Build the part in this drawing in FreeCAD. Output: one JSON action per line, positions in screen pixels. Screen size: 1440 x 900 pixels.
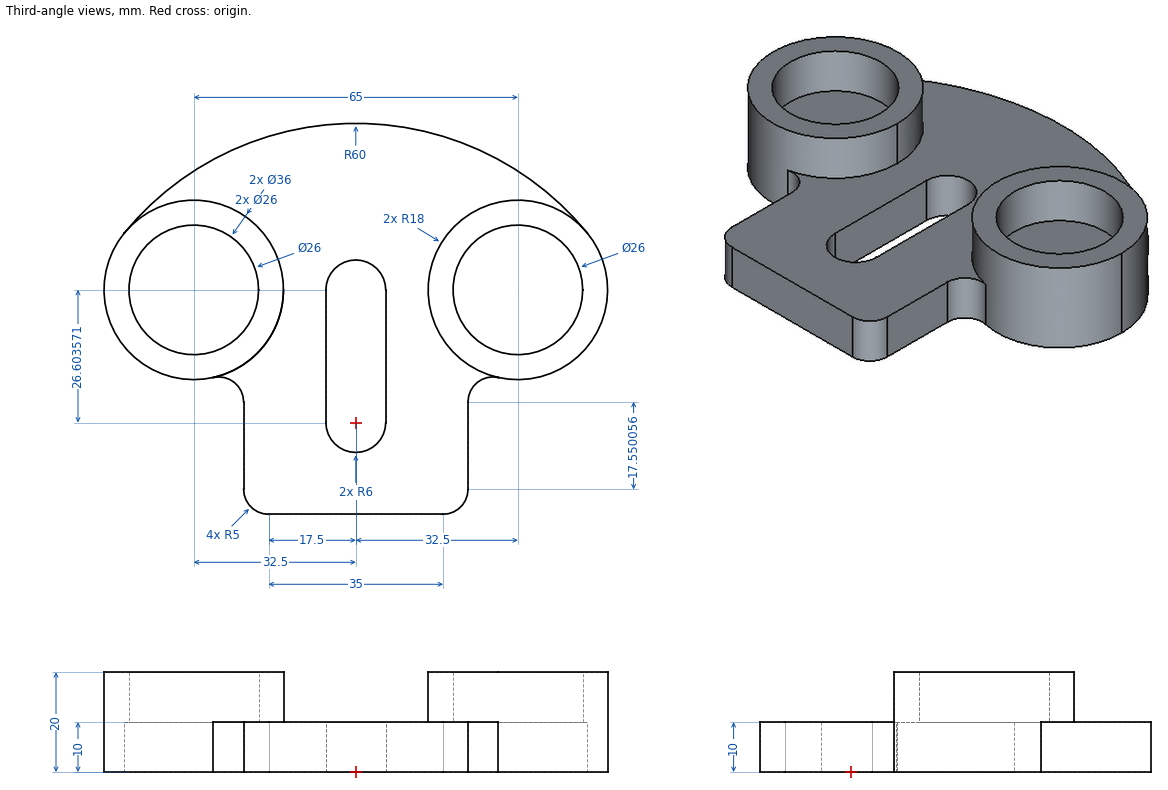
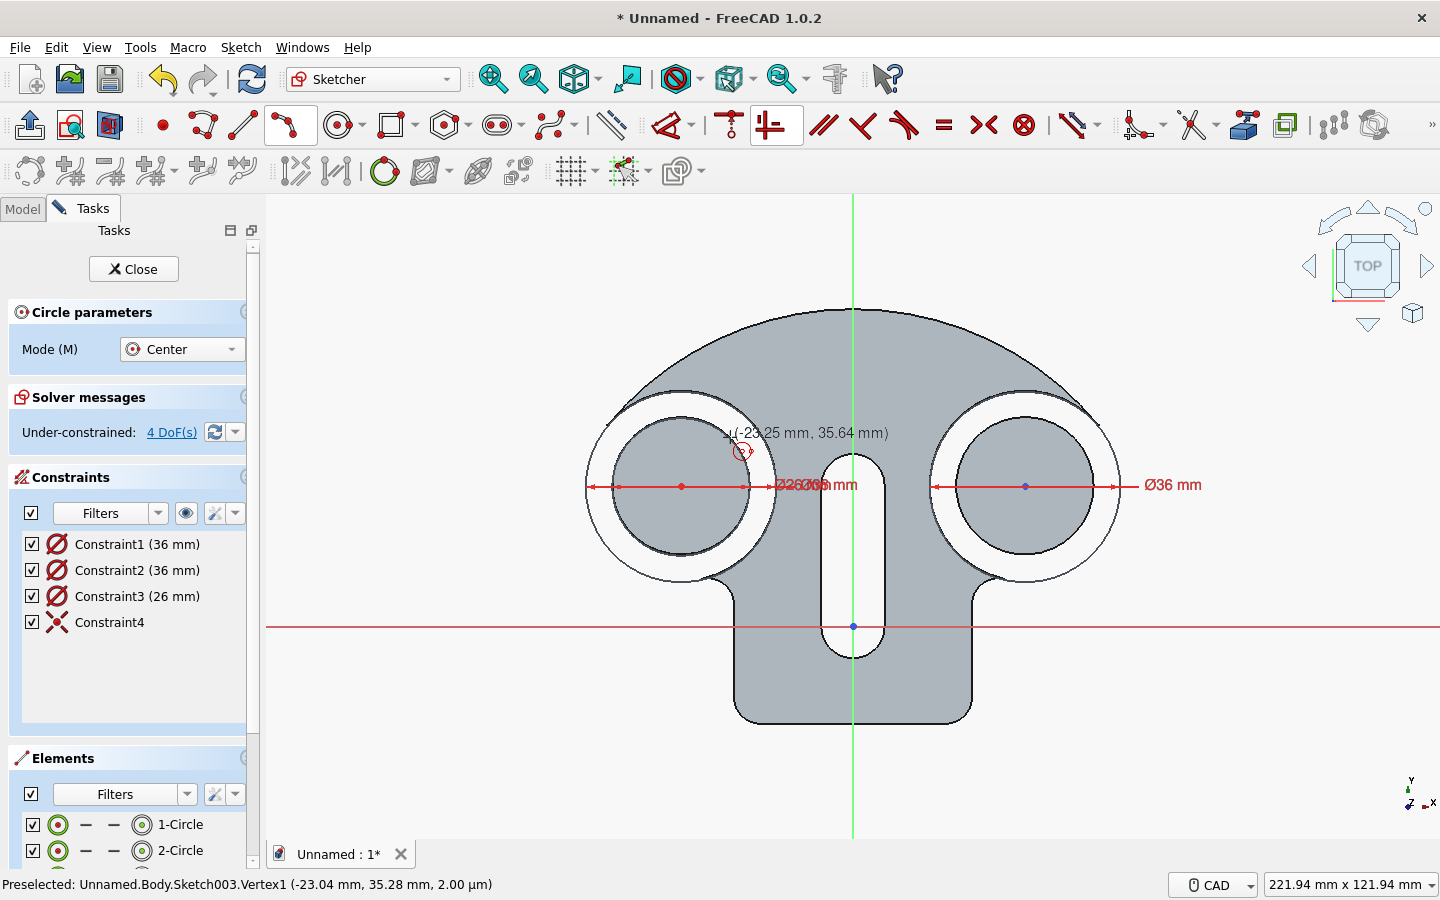
{"action": "left_click", "coordinate": [1025, 487]}
{"action": "mouse_move", "coordinate": [1074, 437]}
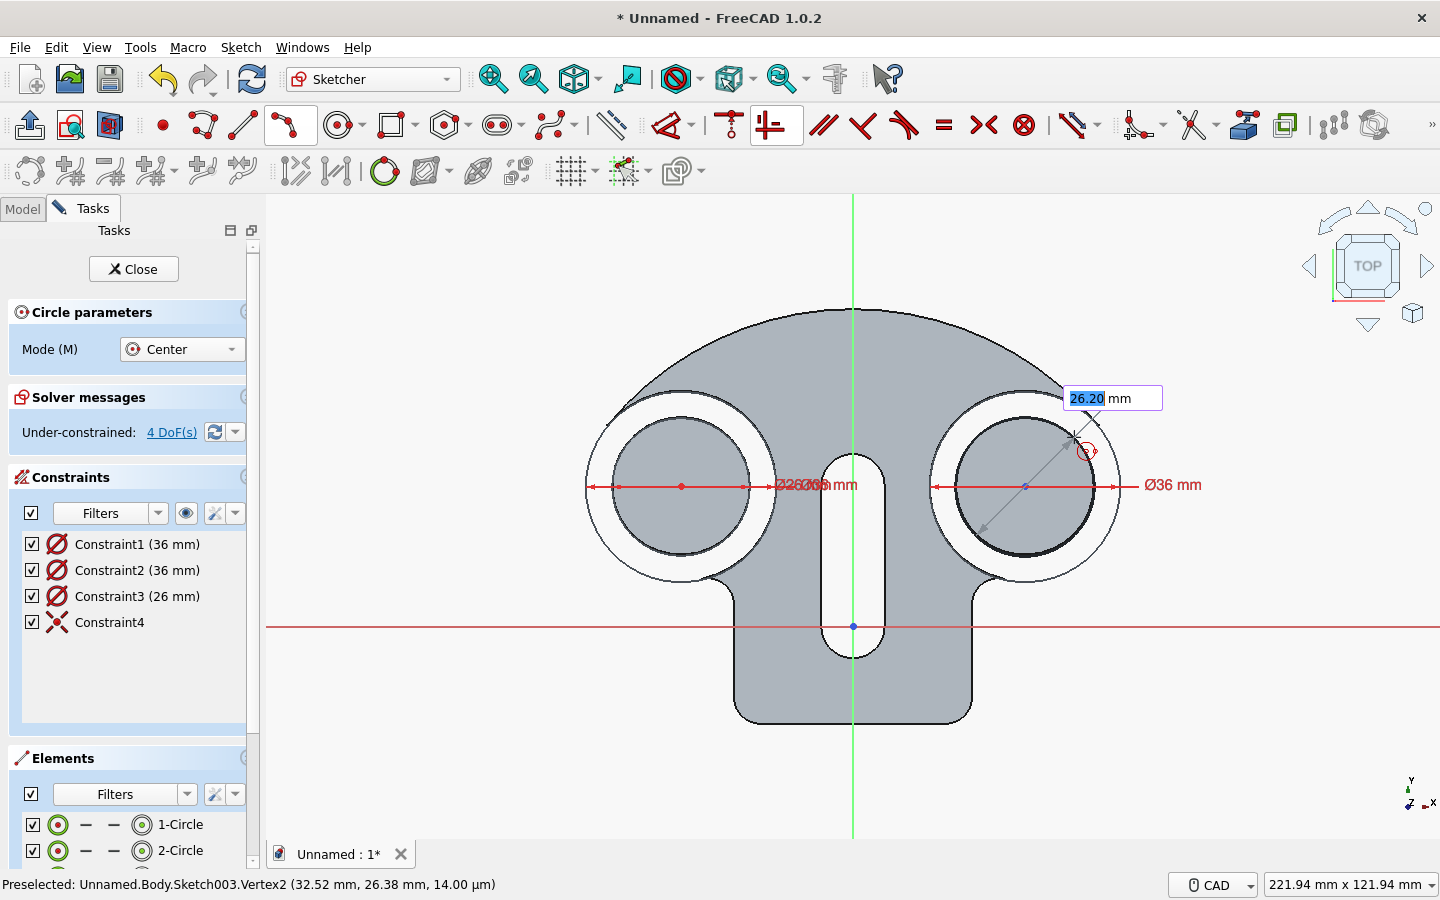
{"action": "type", "text": "26"}
{"action": "key", "text": "Return"}
{"action": "key", "text": "Escape"}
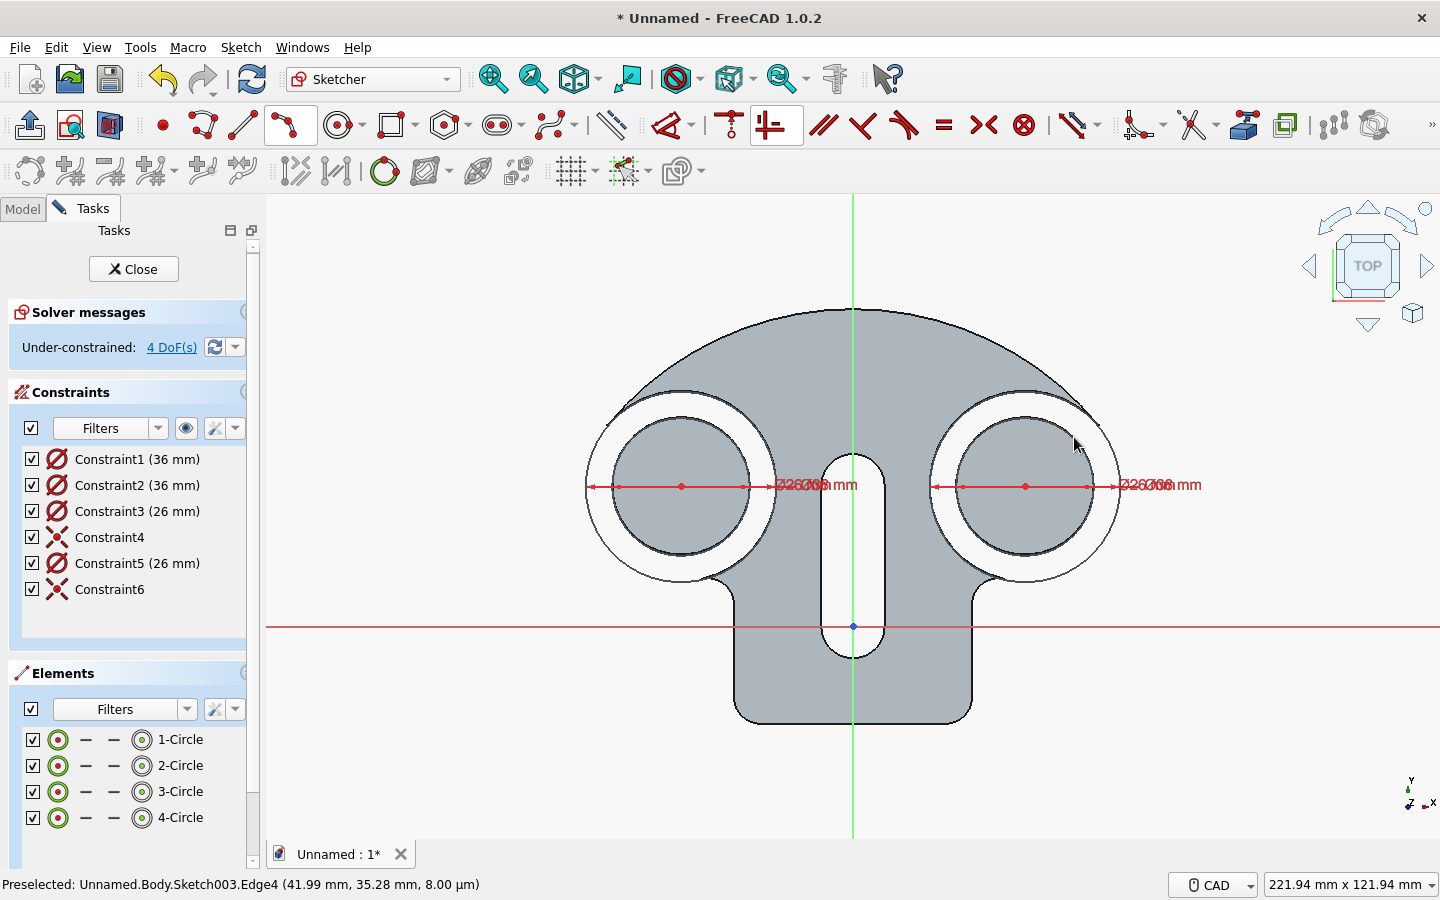
{"action": "left_click", "coordinate": [681, 487]}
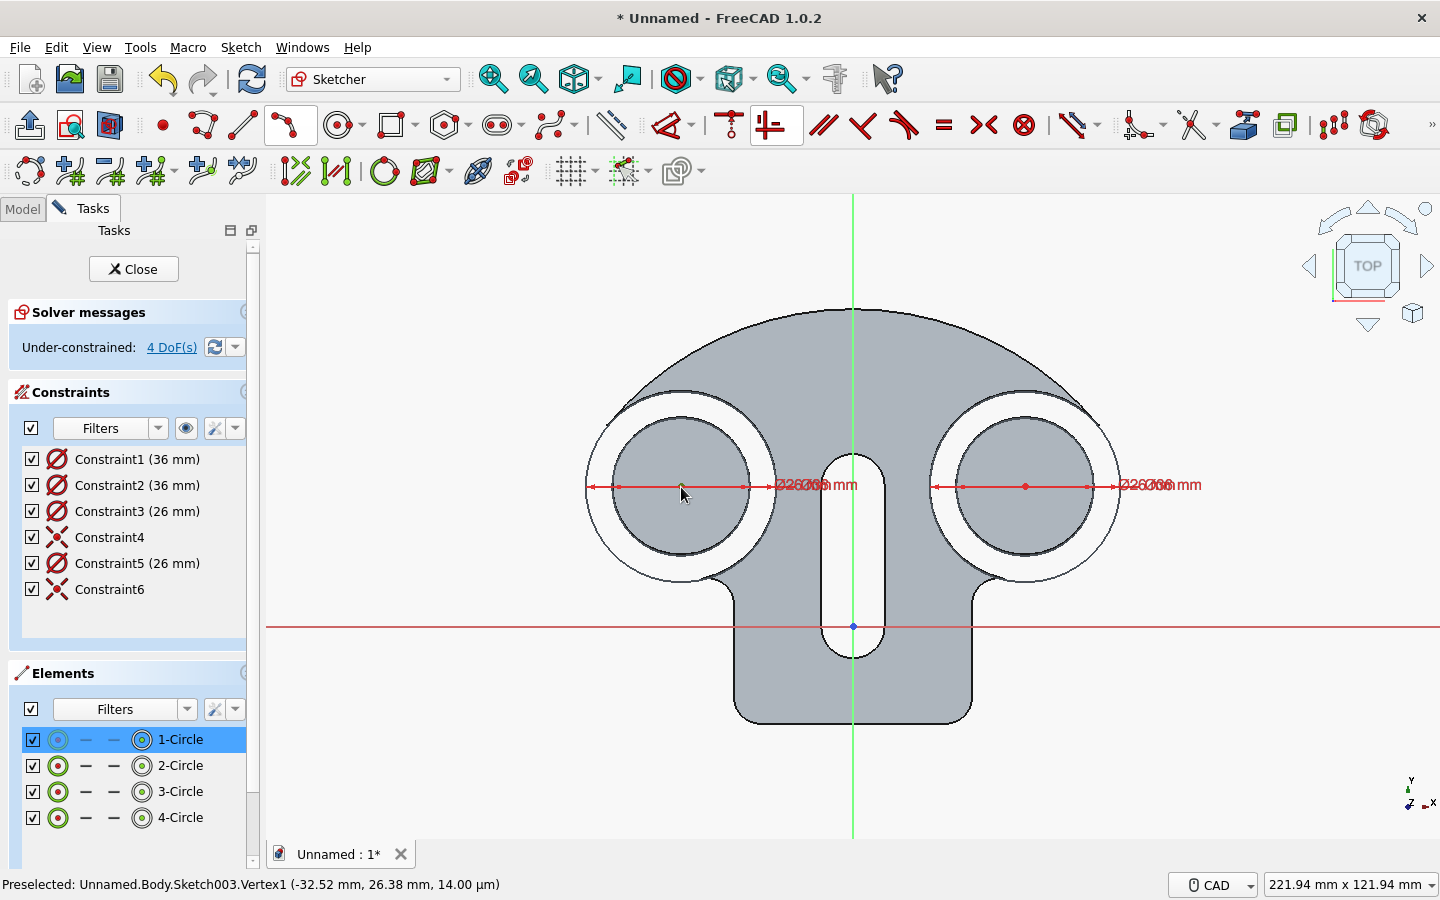
{"action": "left_click", "coordinate": [1025, 487]}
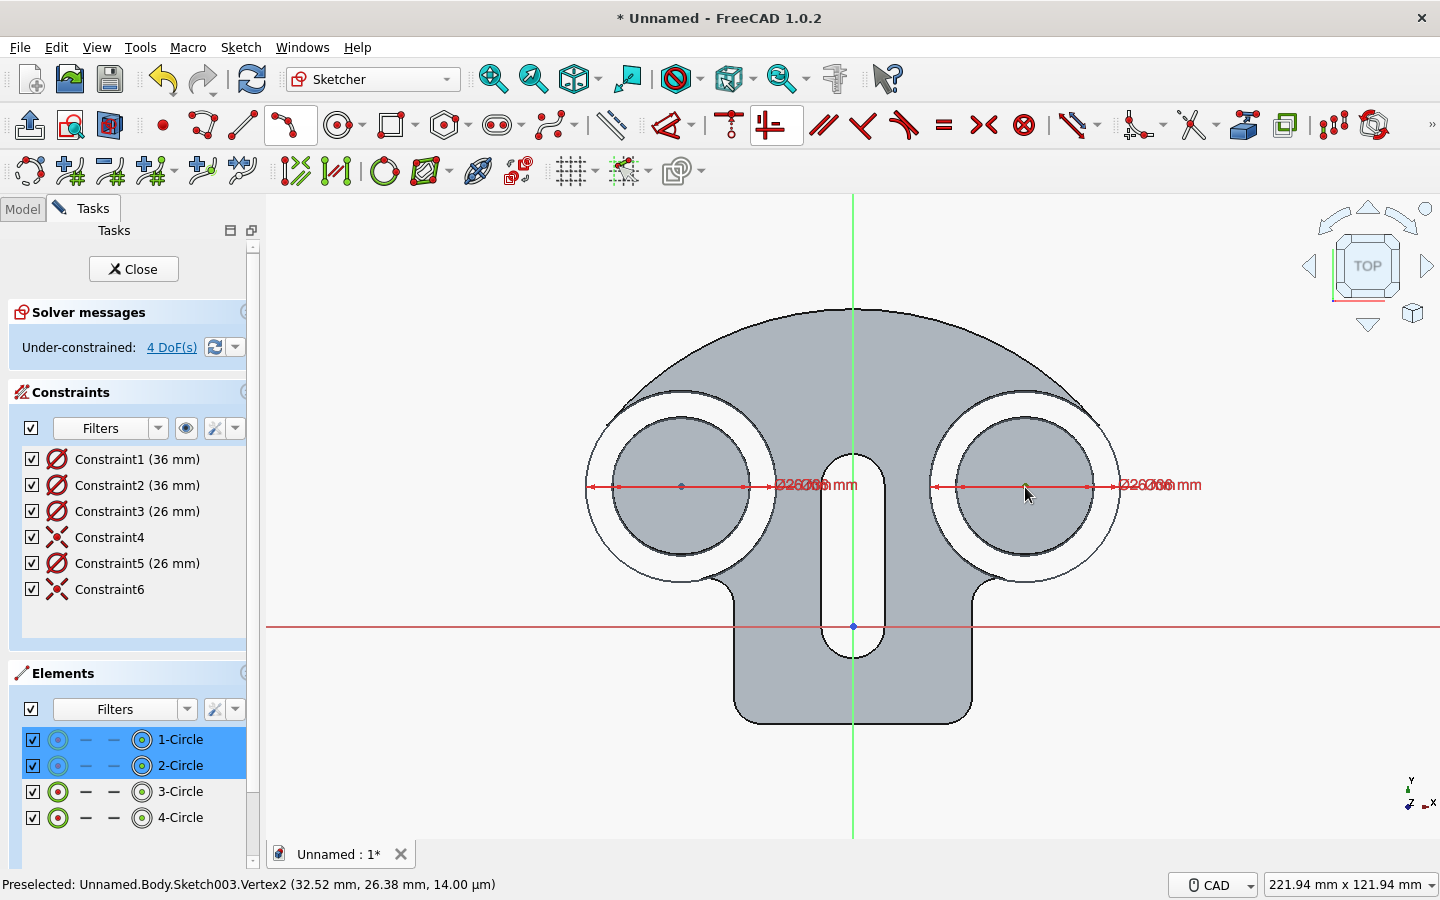
{"action": "key", "text": "h"}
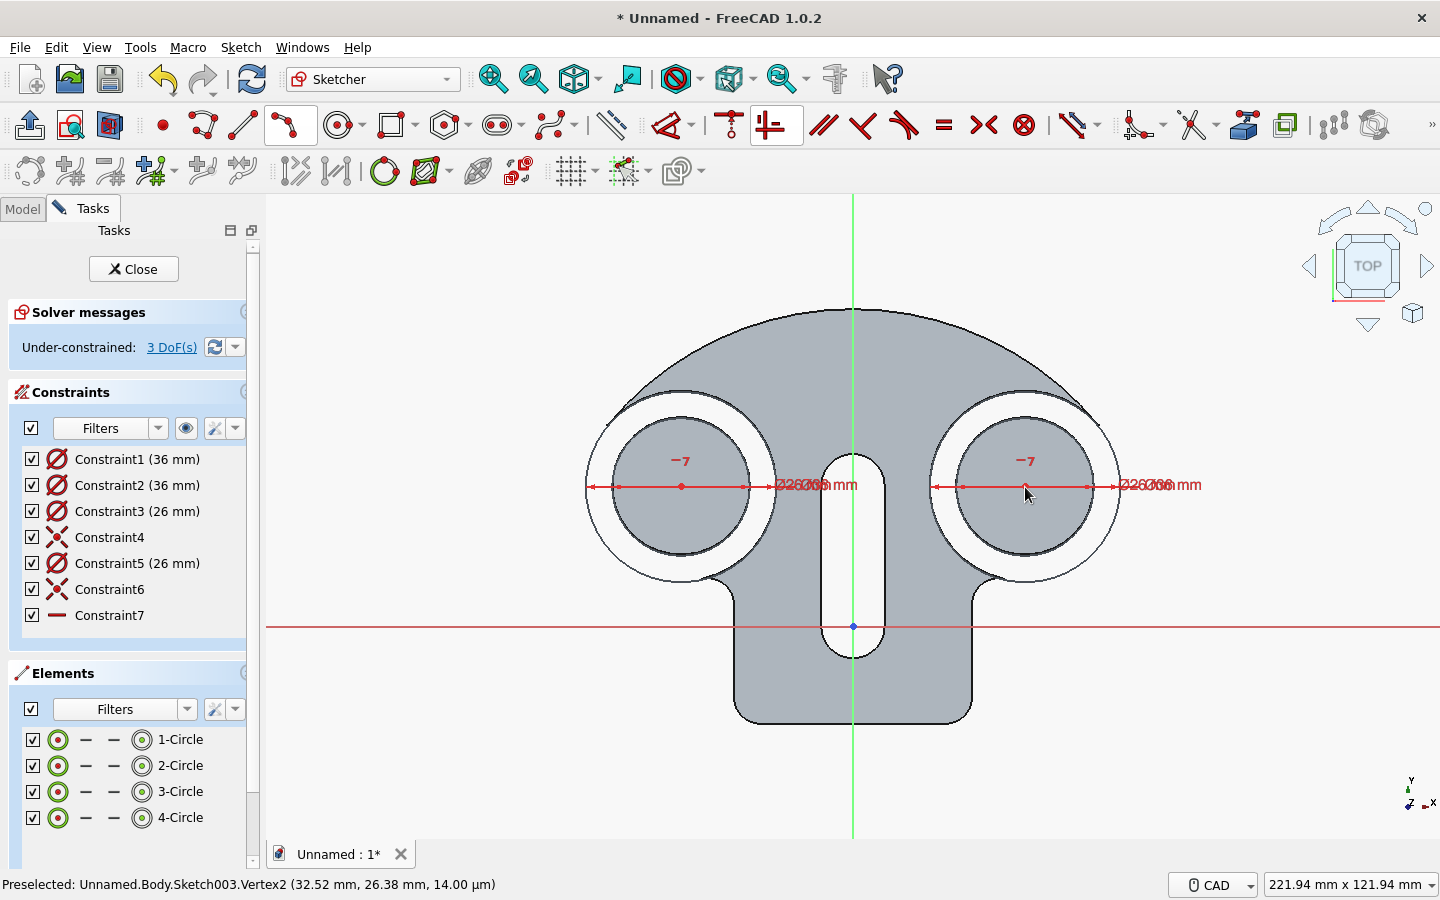
{"action": "left_click", "coordinate": [666, 126]}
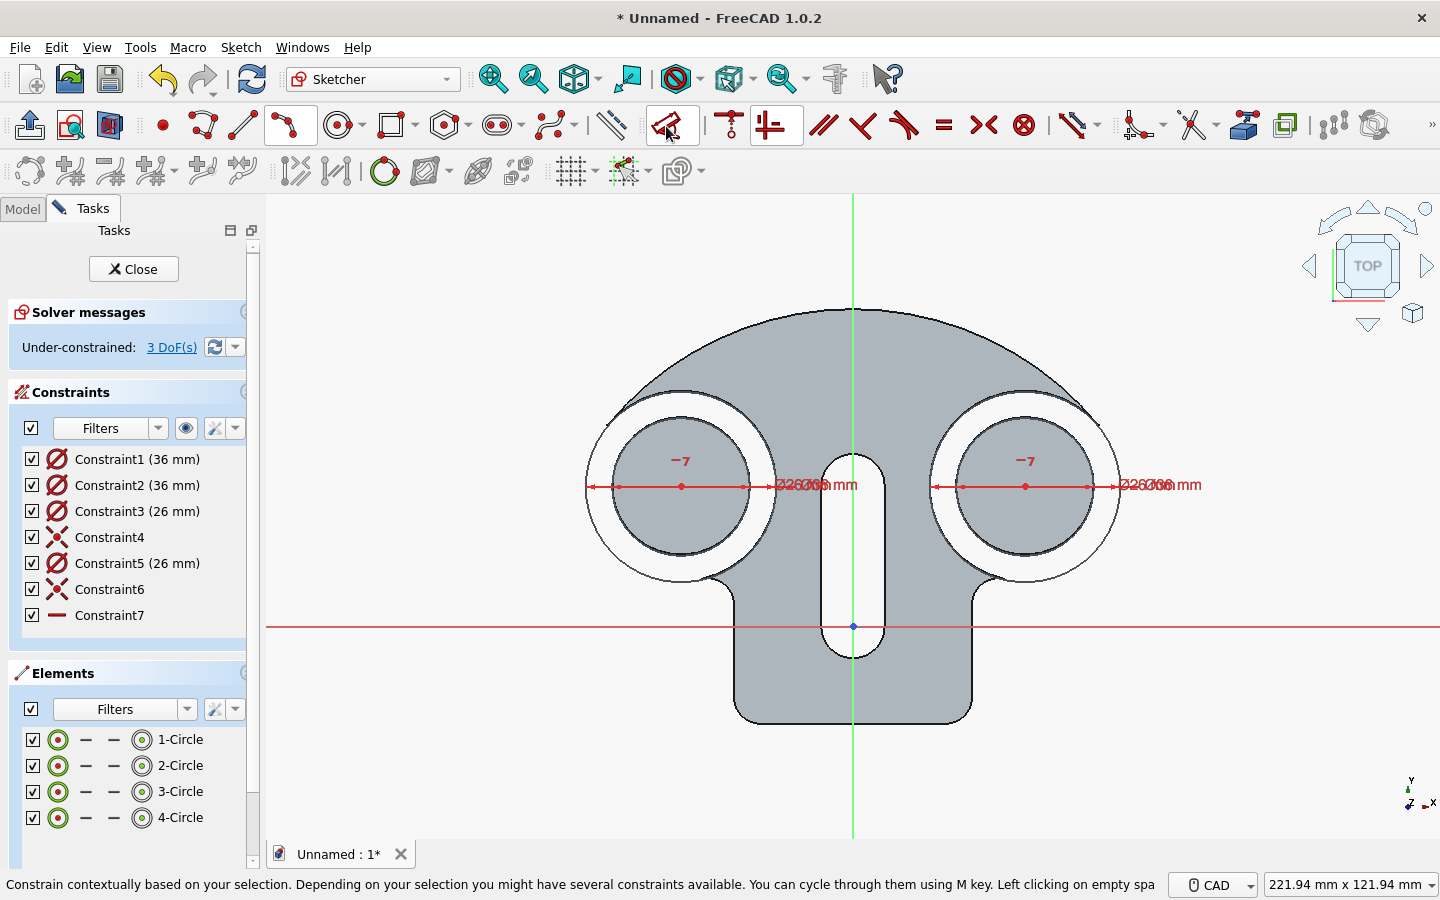
{"action": "left_click", "coordinate": [681, 487]}